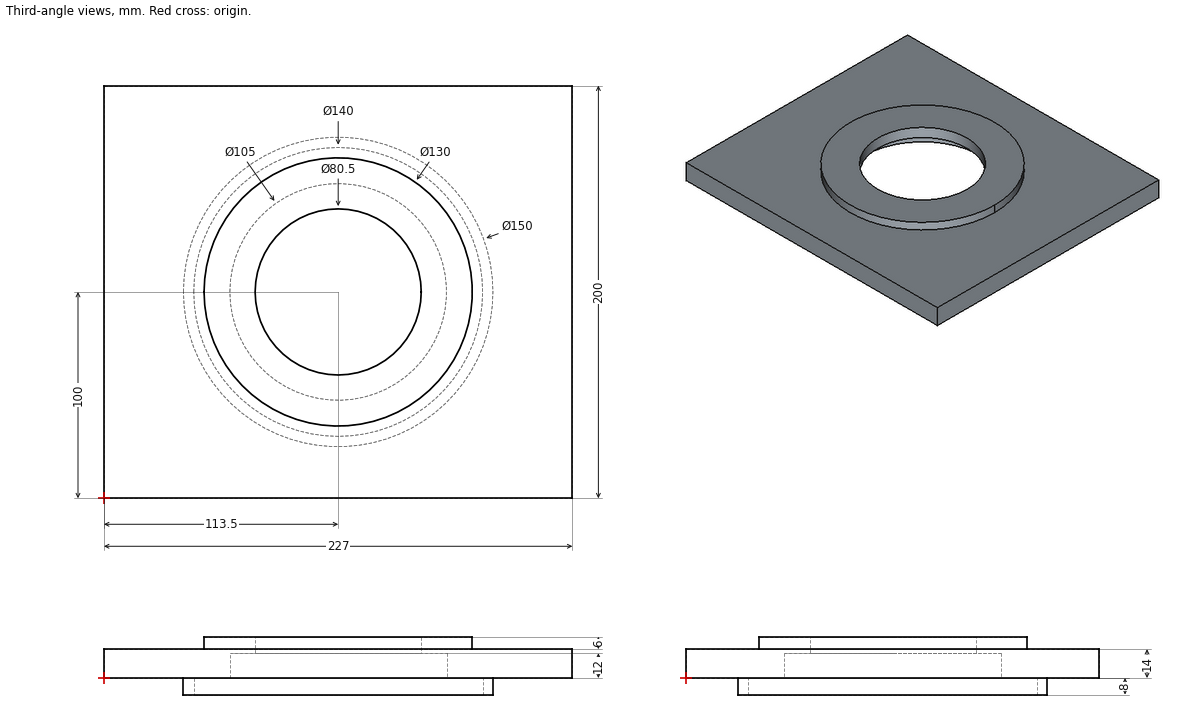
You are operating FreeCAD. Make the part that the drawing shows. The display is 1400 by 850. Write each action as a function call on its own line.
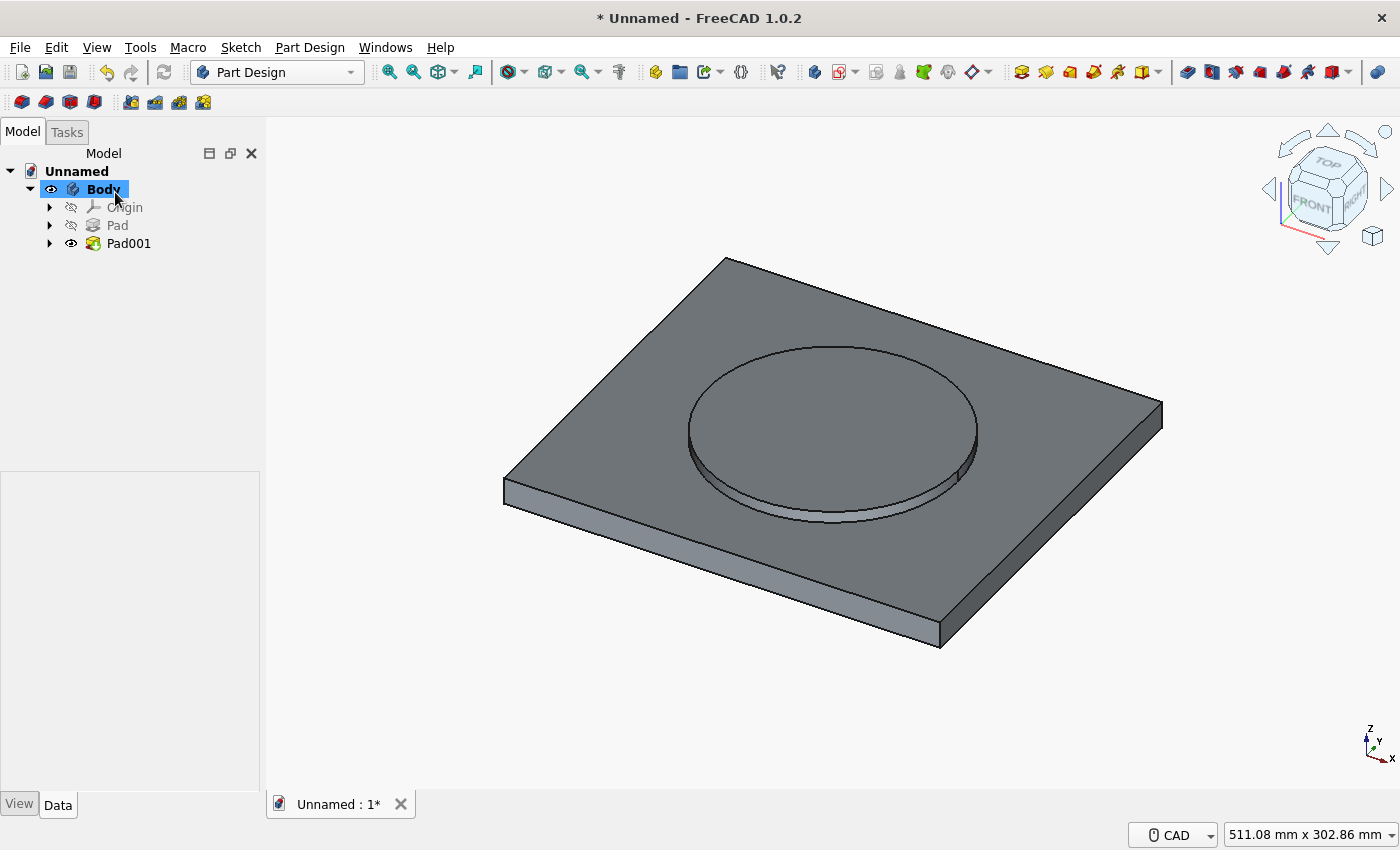
click(840, 72)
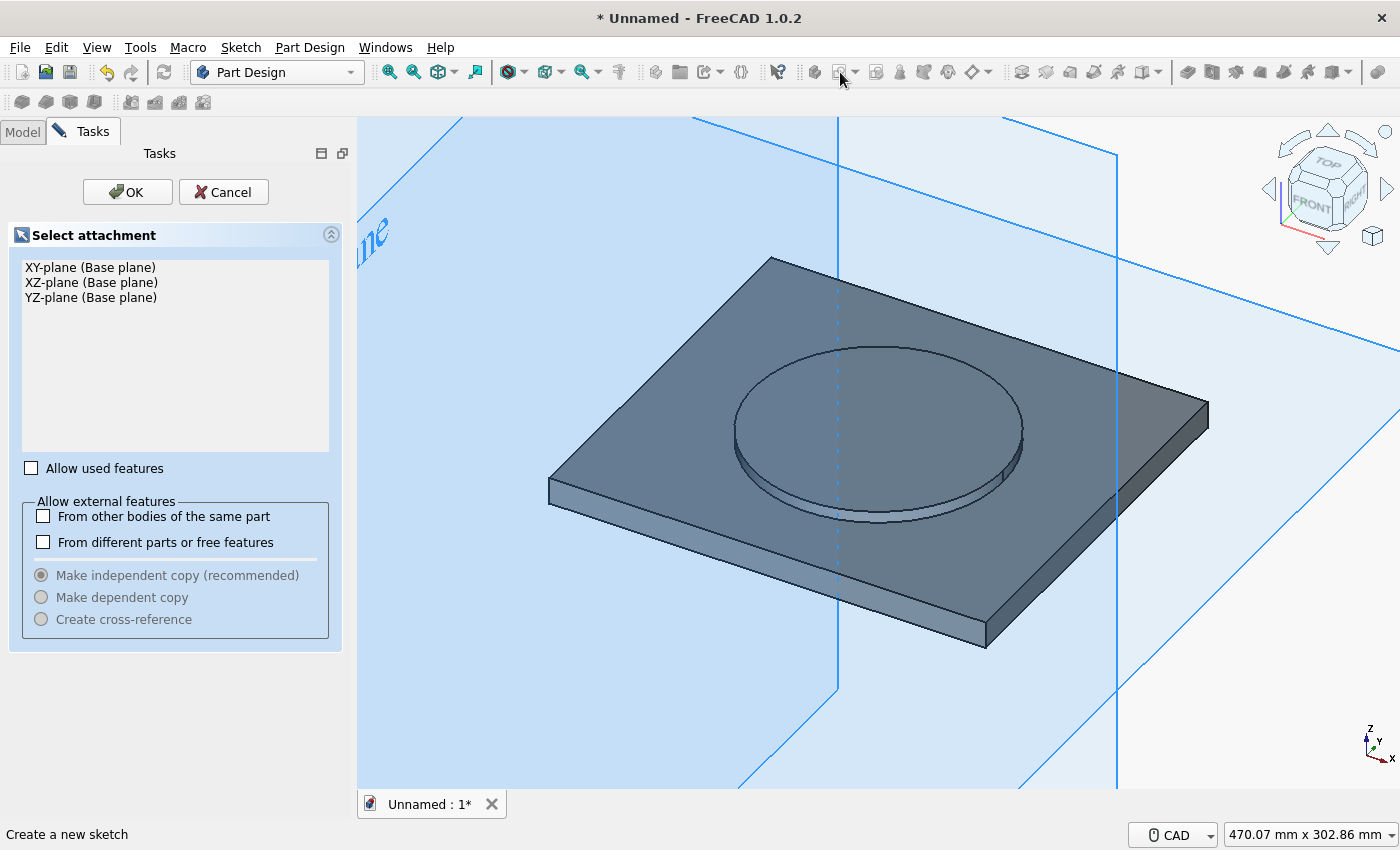
click(82, 268)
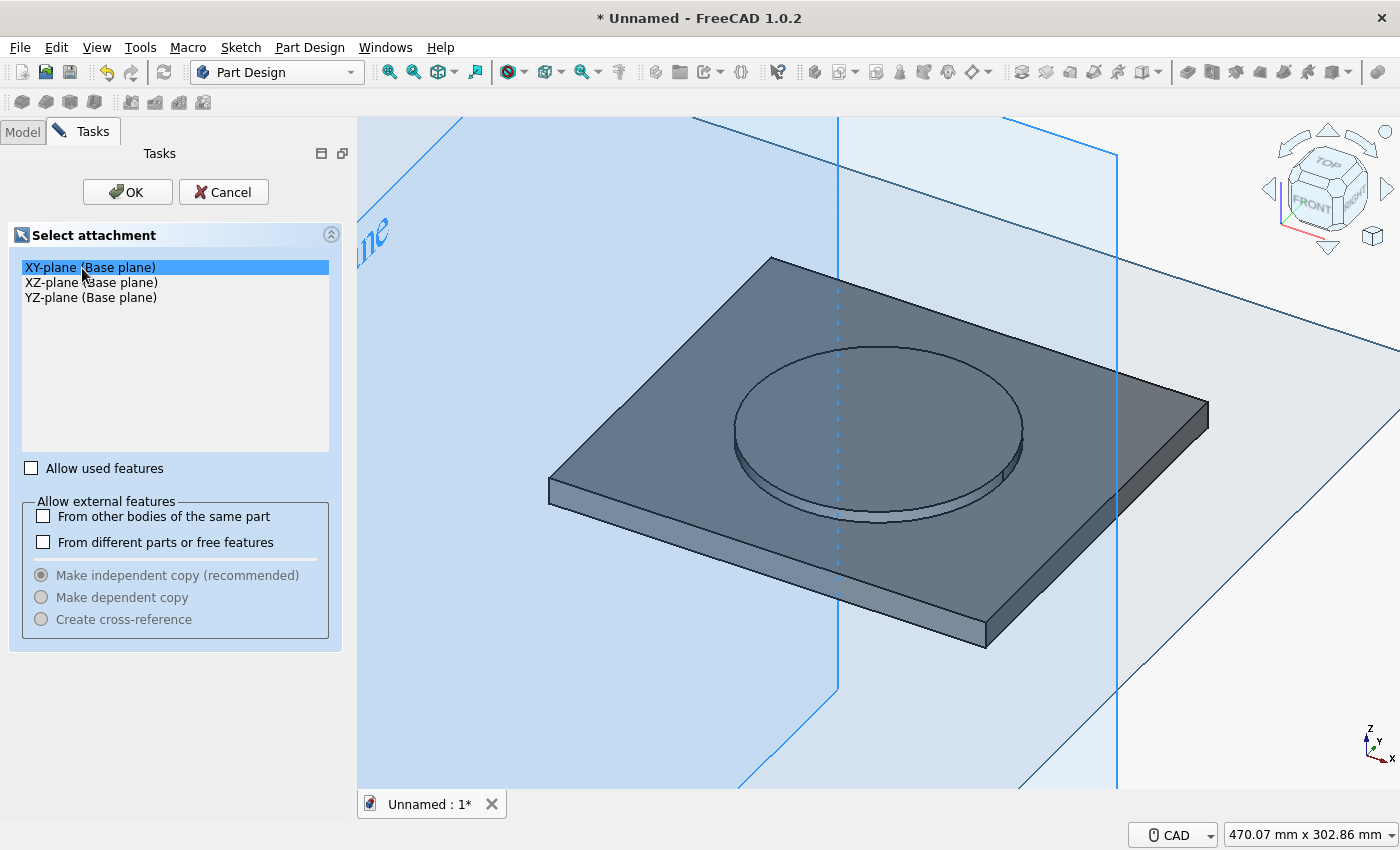
click(128, 192)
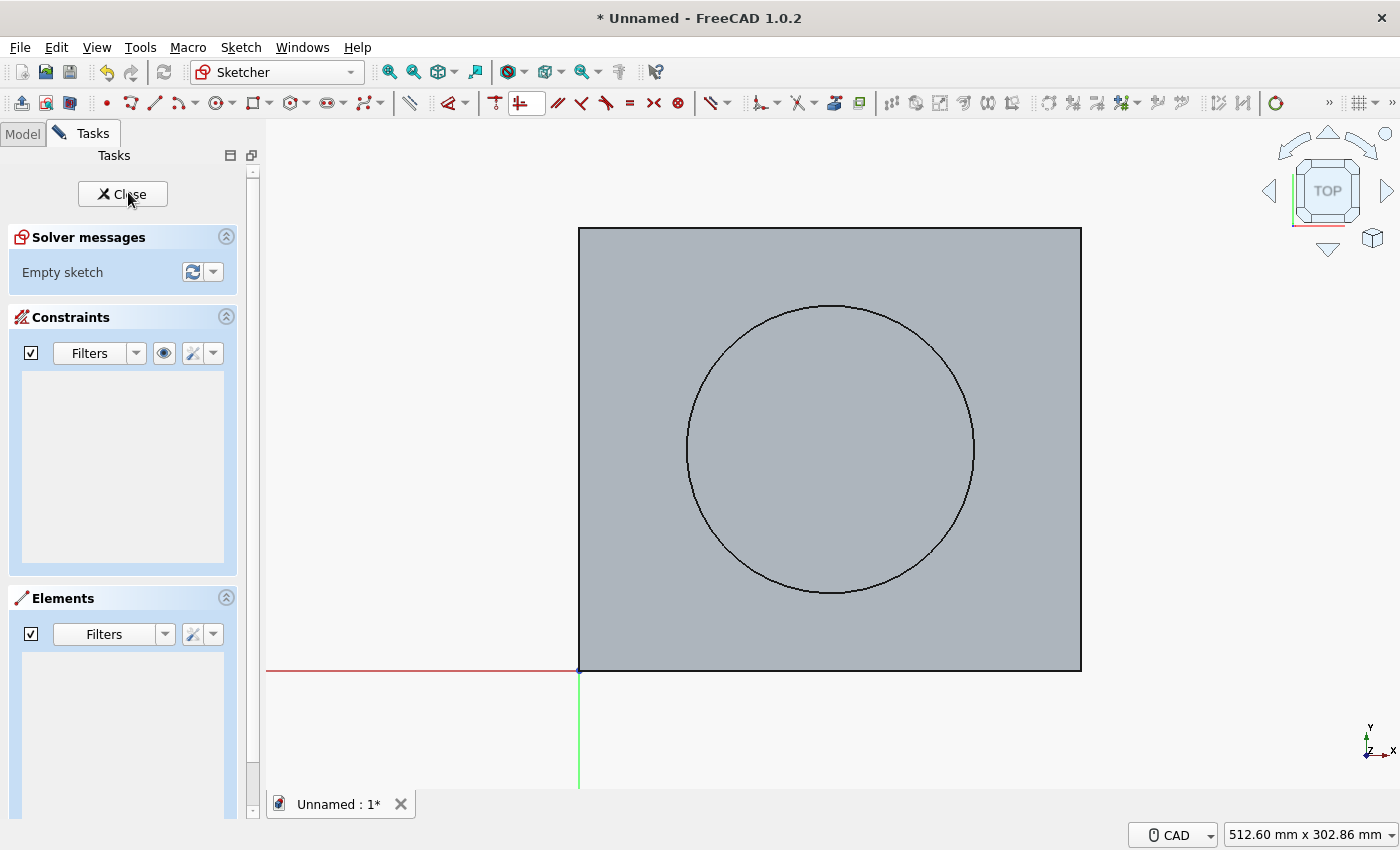
key(q)
key(s)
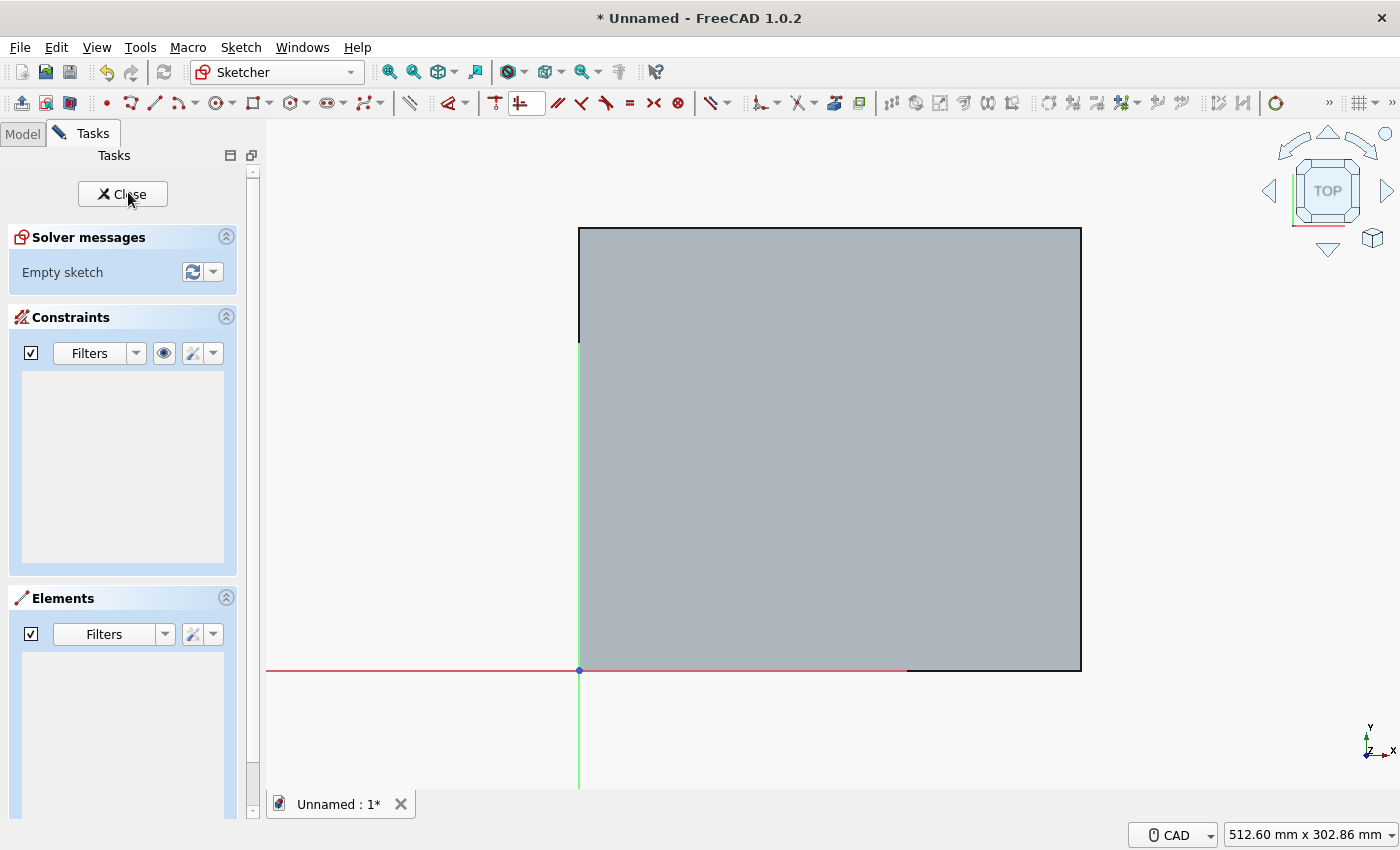
key(g)
key(c)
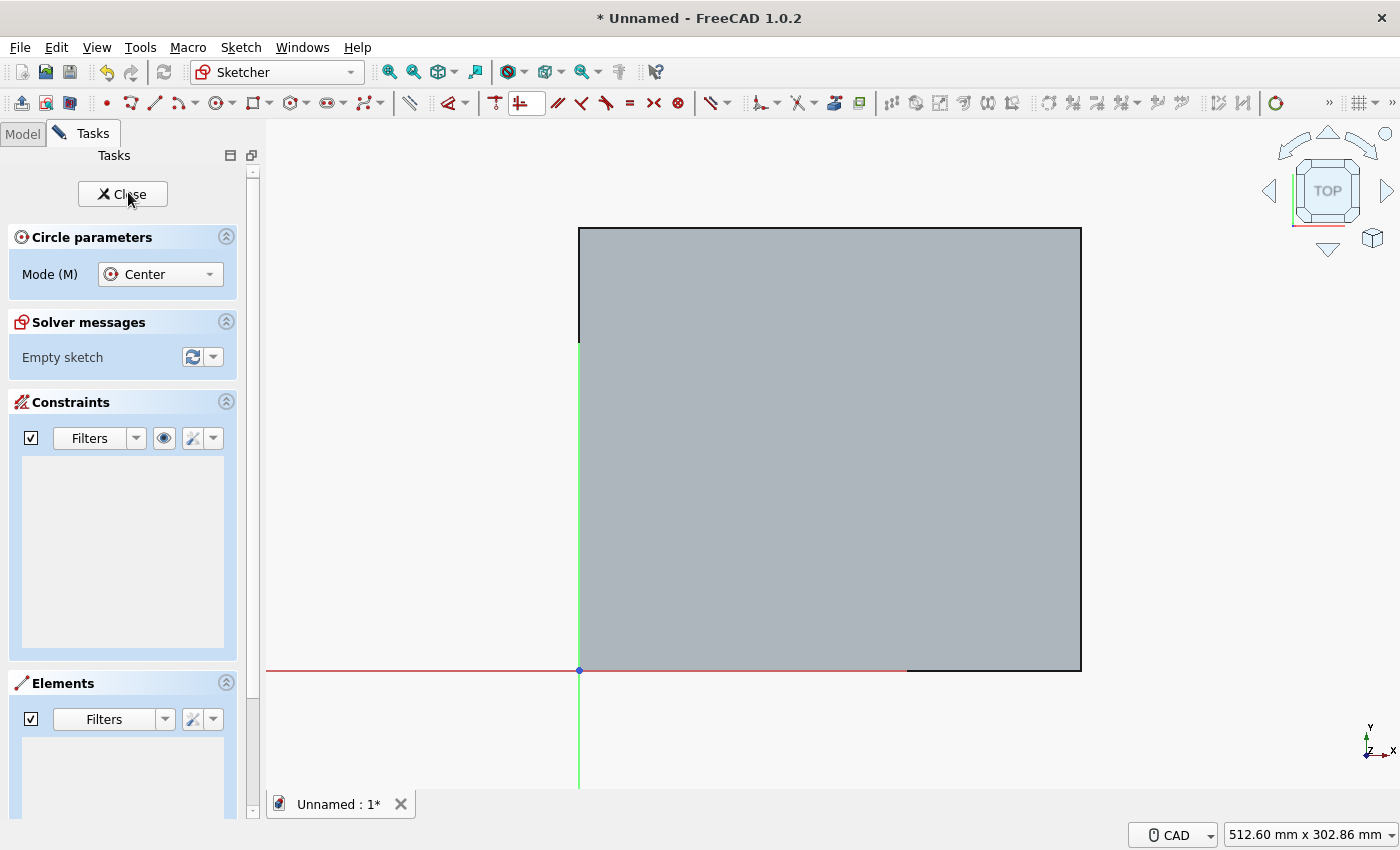
click(830, 449)
click(948, 332)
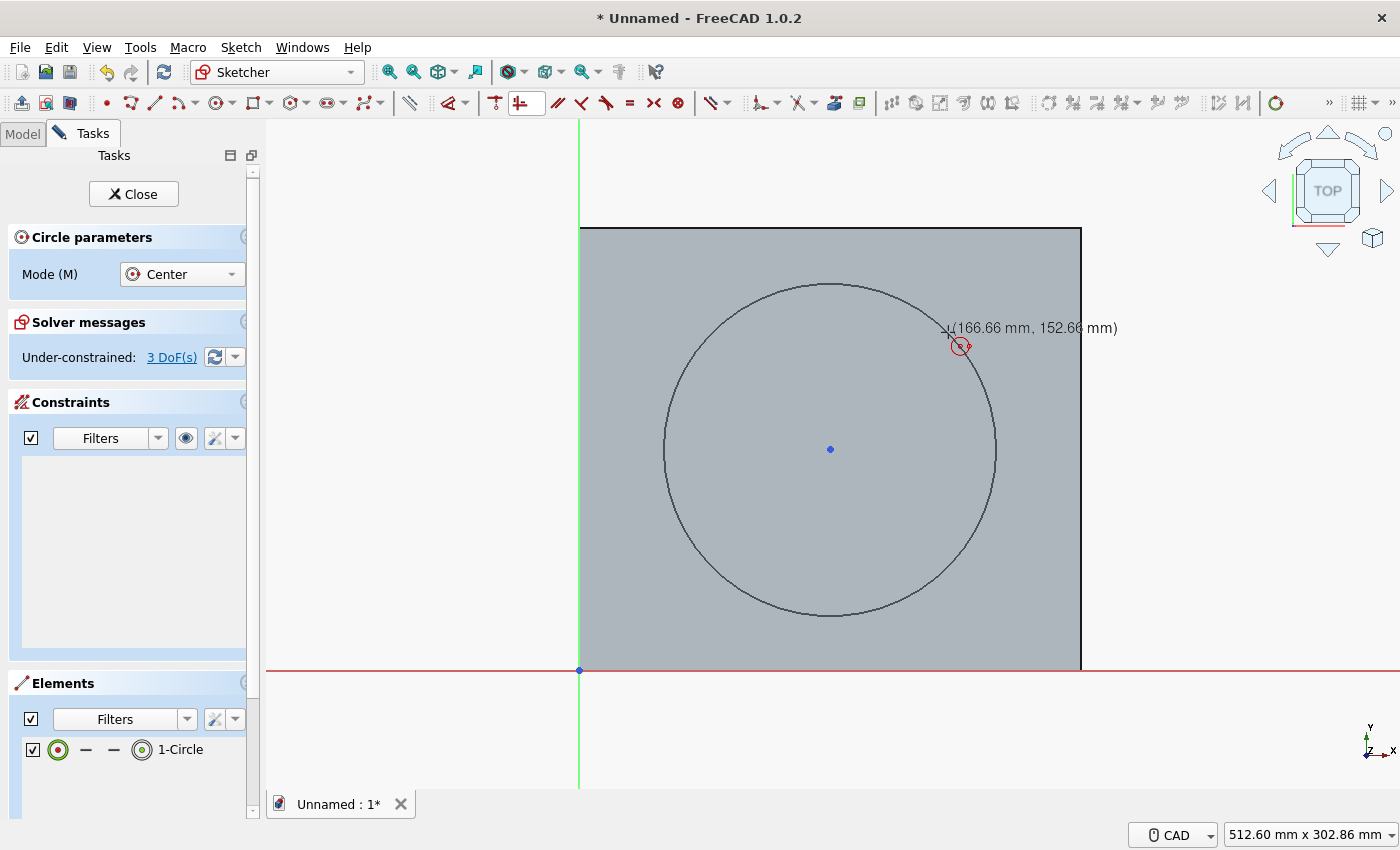
click(830, 450)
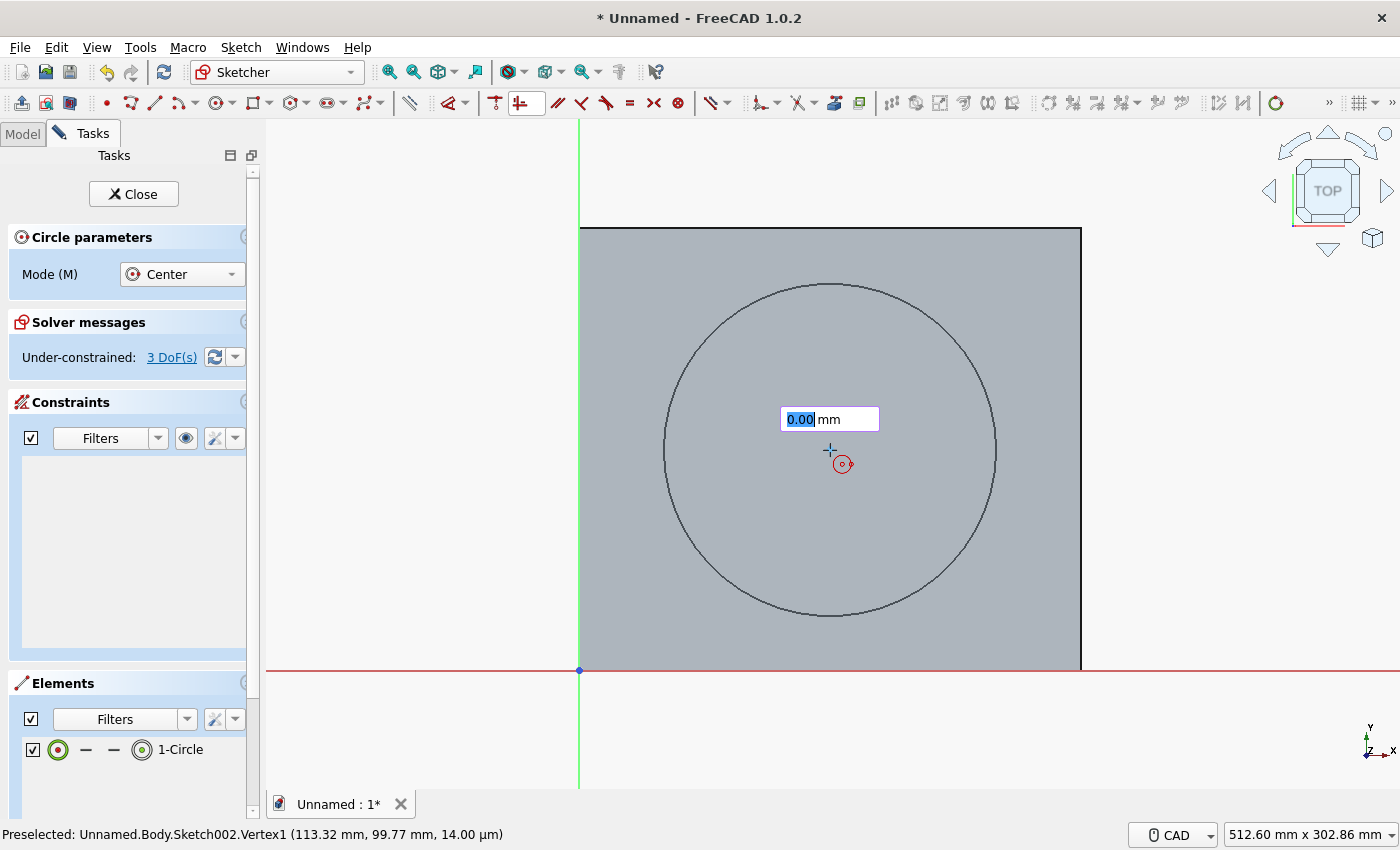
scroll(940, 340, up, 2)